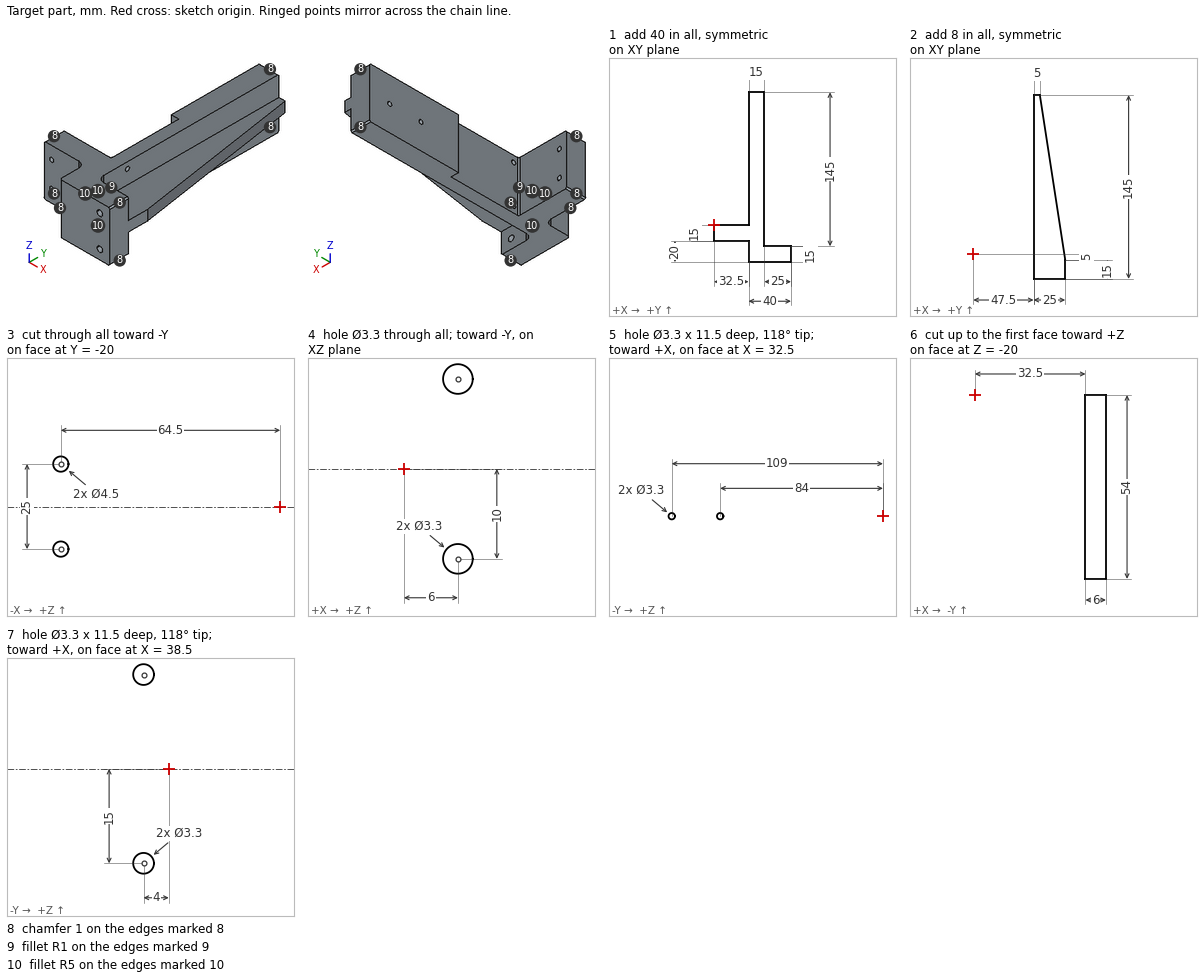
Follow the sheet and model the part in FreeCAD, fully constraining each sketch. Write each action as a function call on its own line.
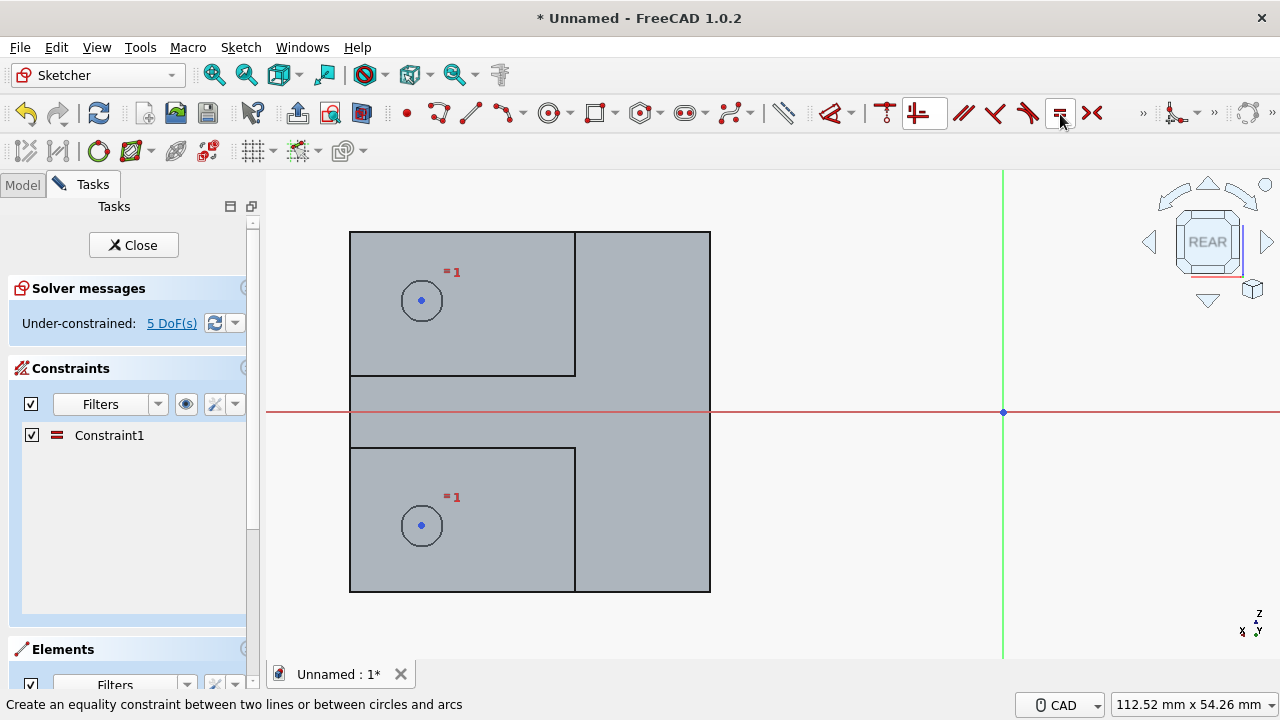
click(422, 301)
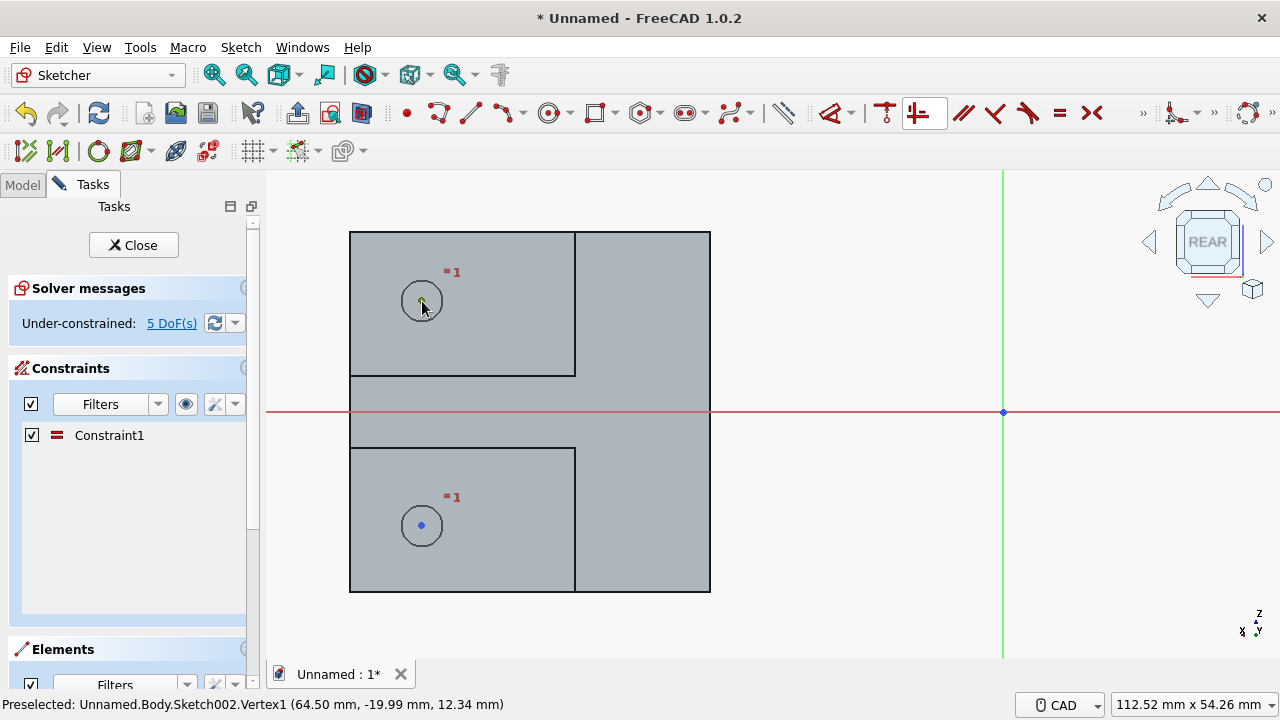
click(422, 526)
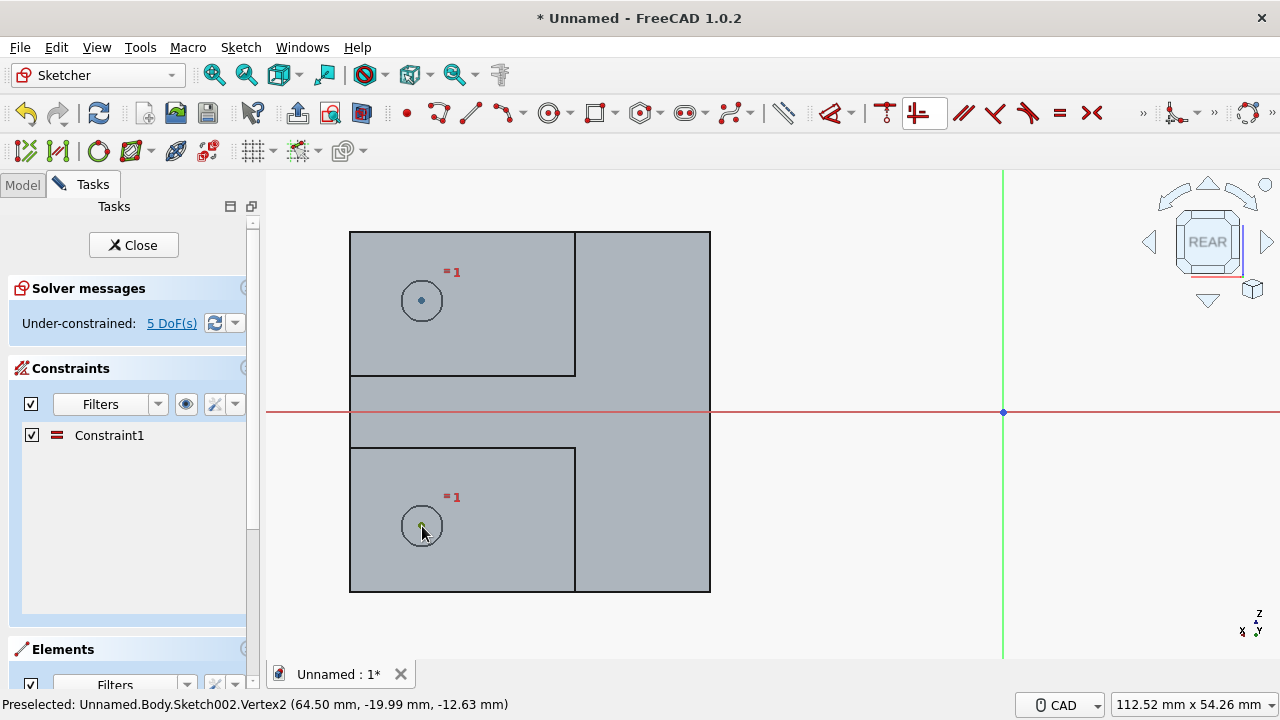
click(353, 412)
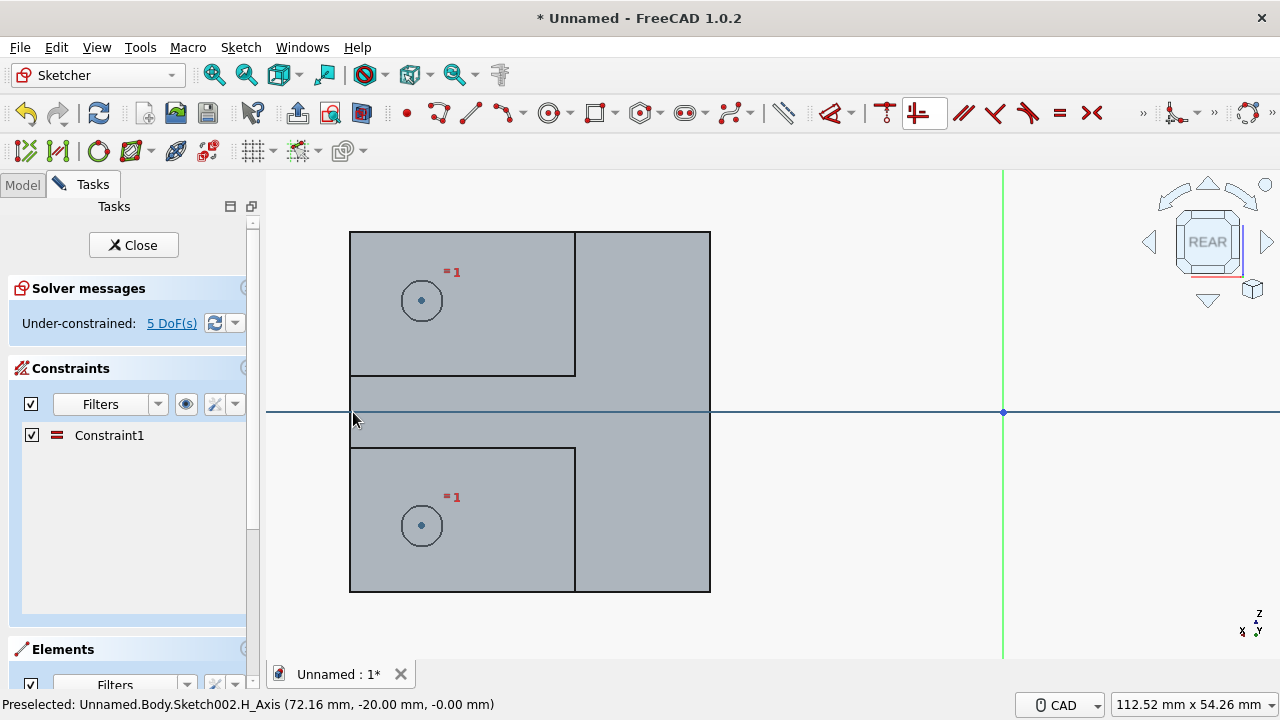
key(s)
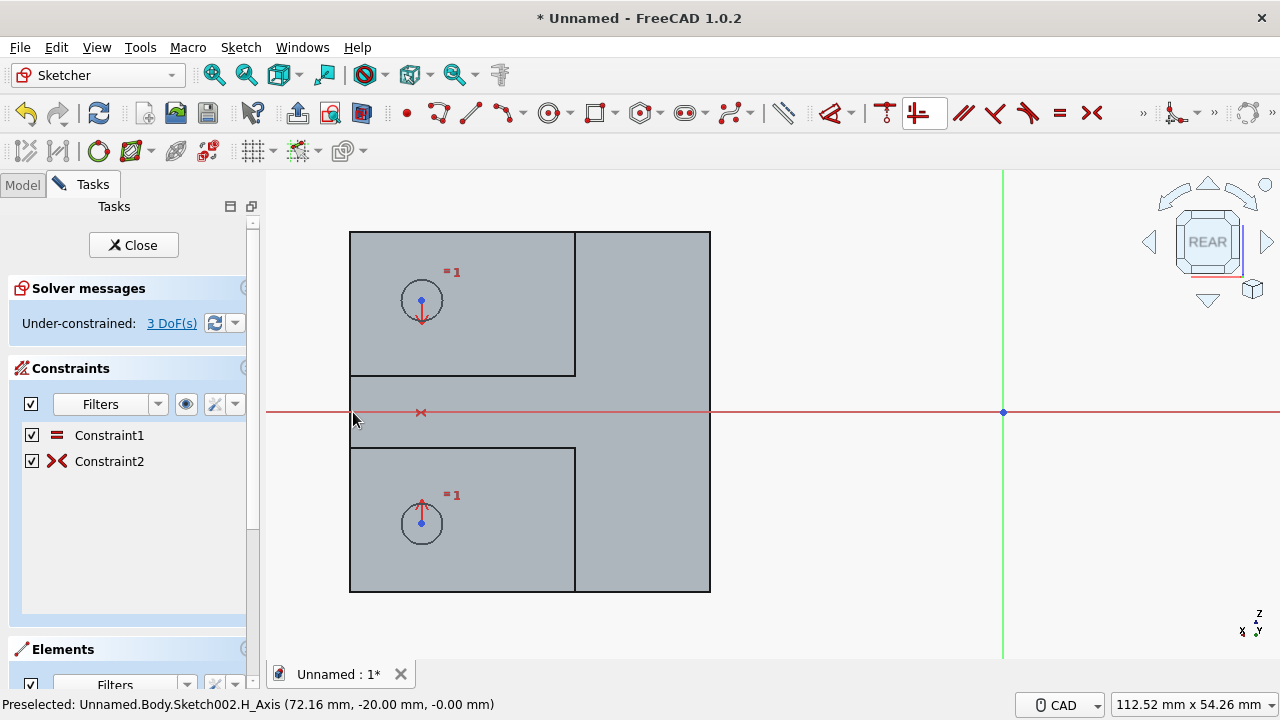
click(830, 114)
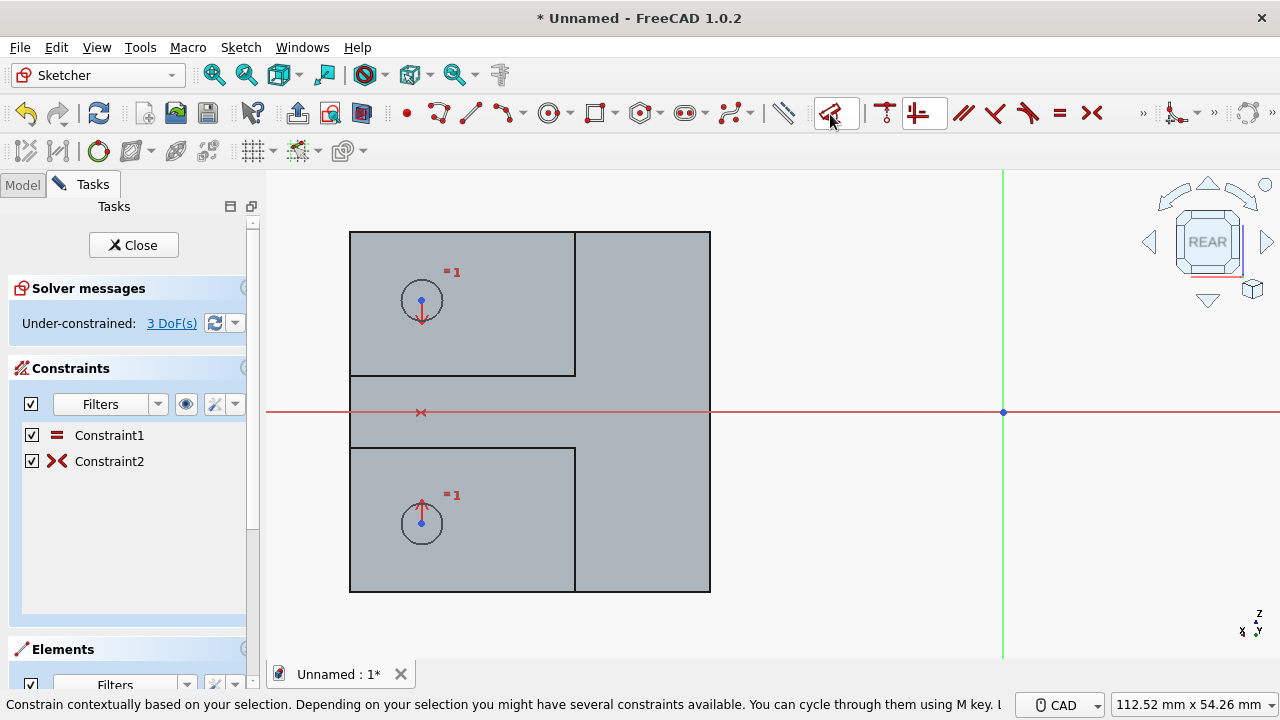
click(436, 286)
click(458, 263)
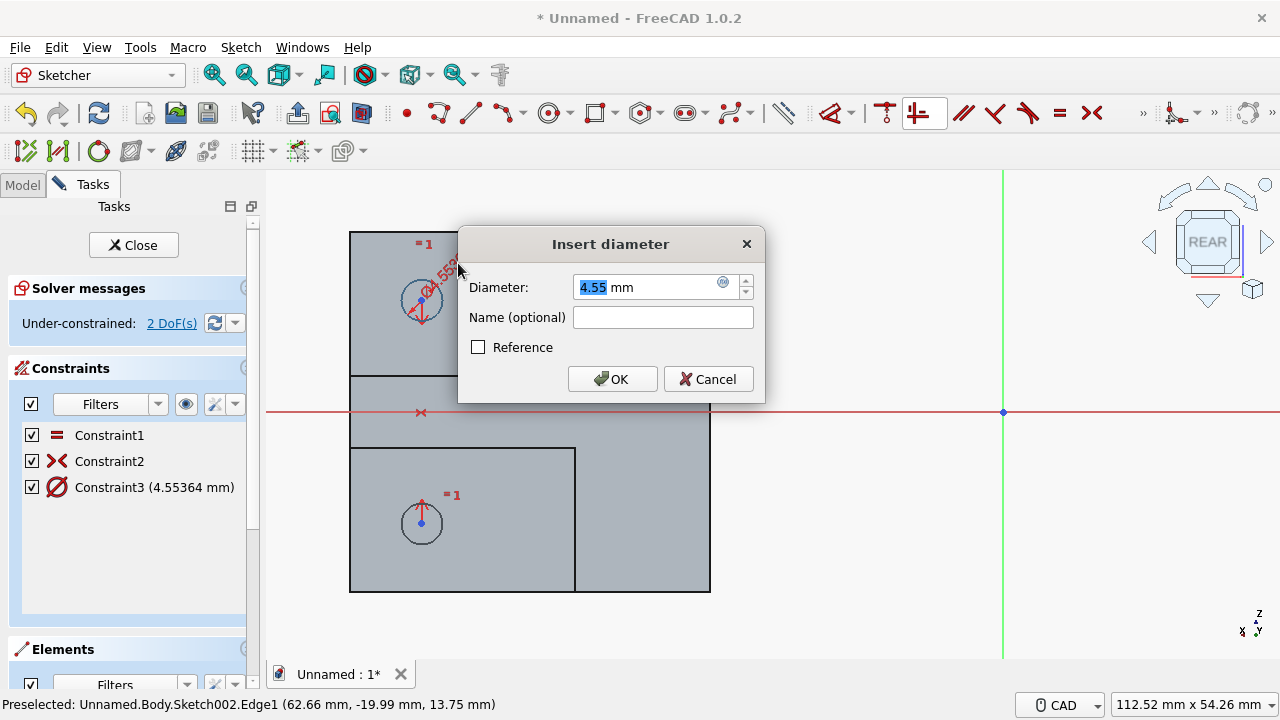
text(4.5)
key(Return)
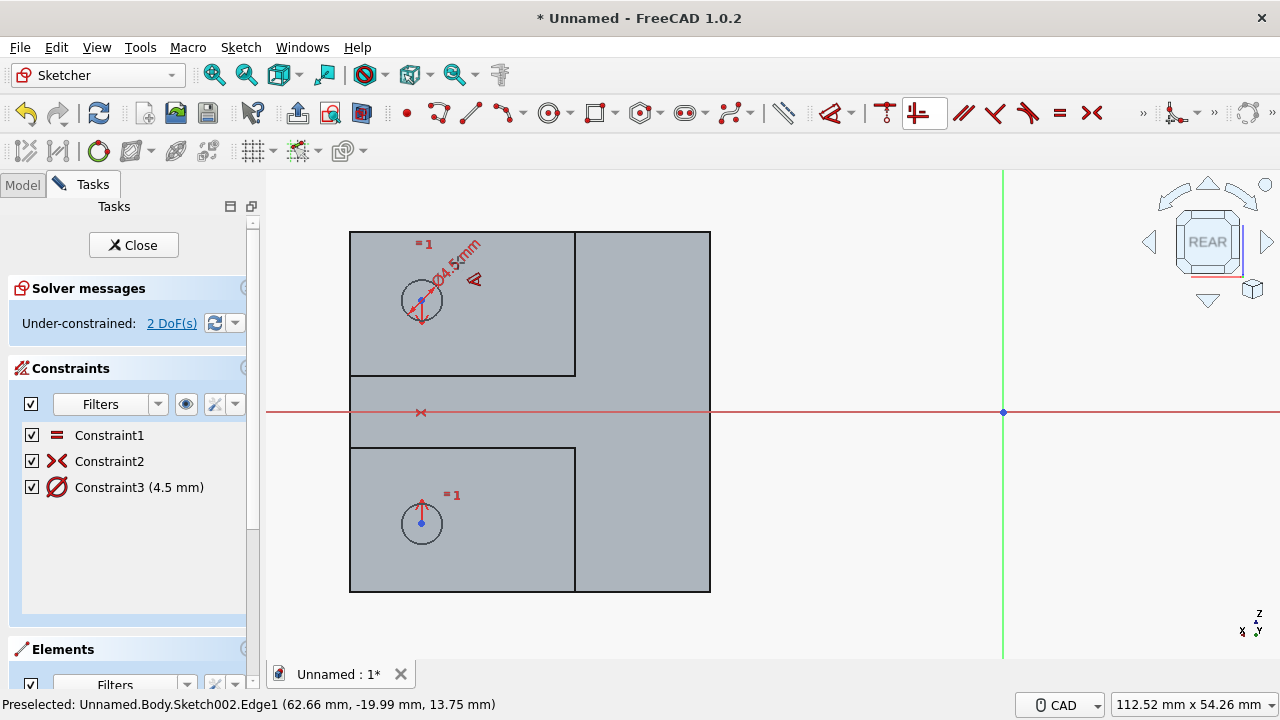
click(422, 300)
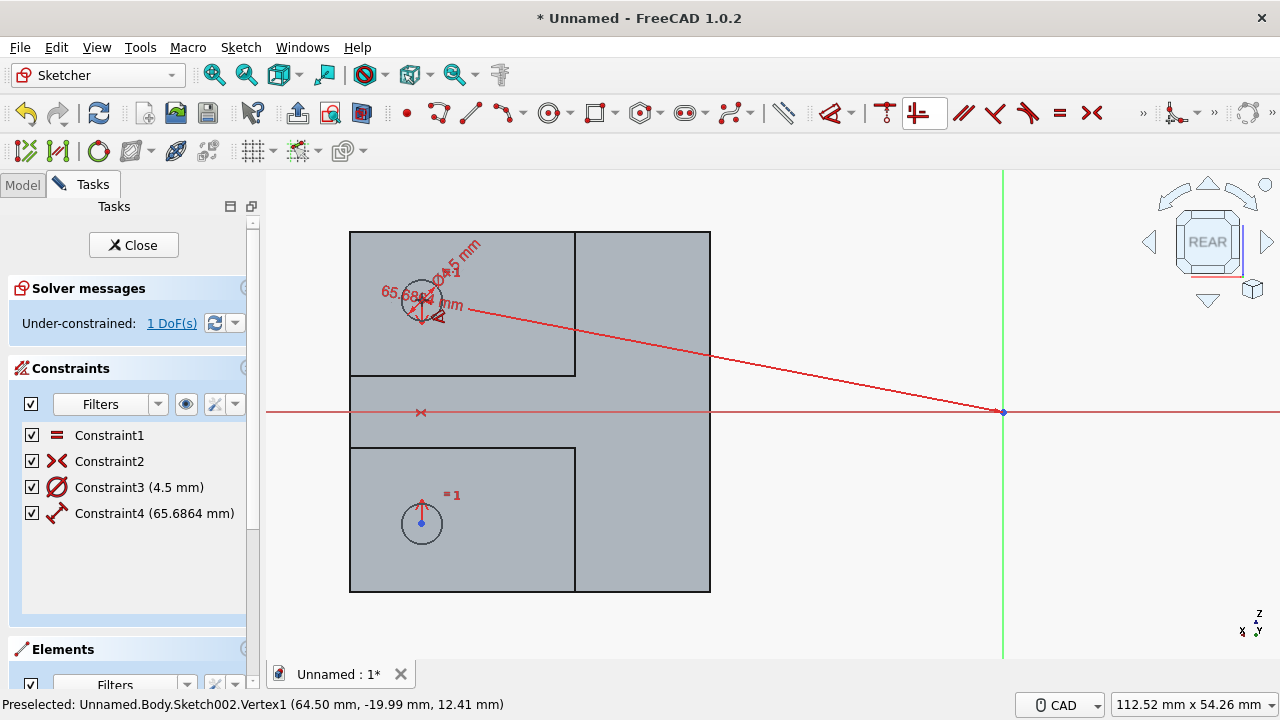
click(422, 524)
click(388, 361)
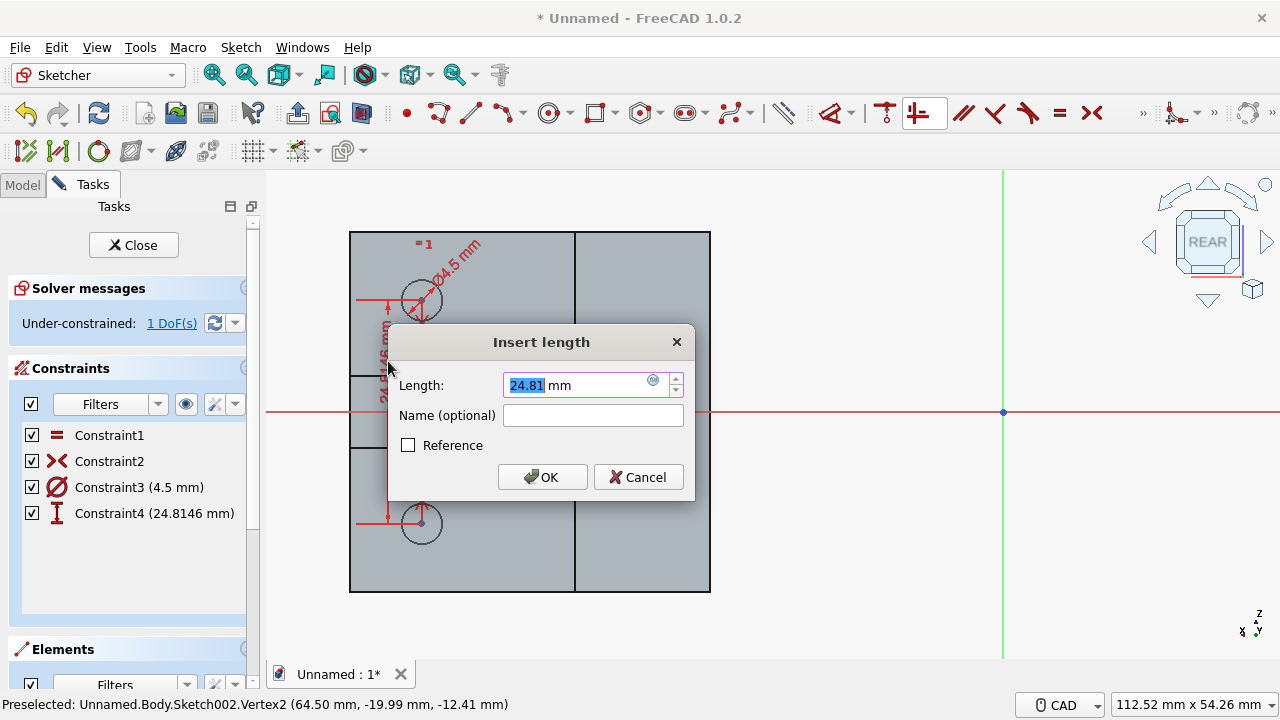
text(25)
key(Return)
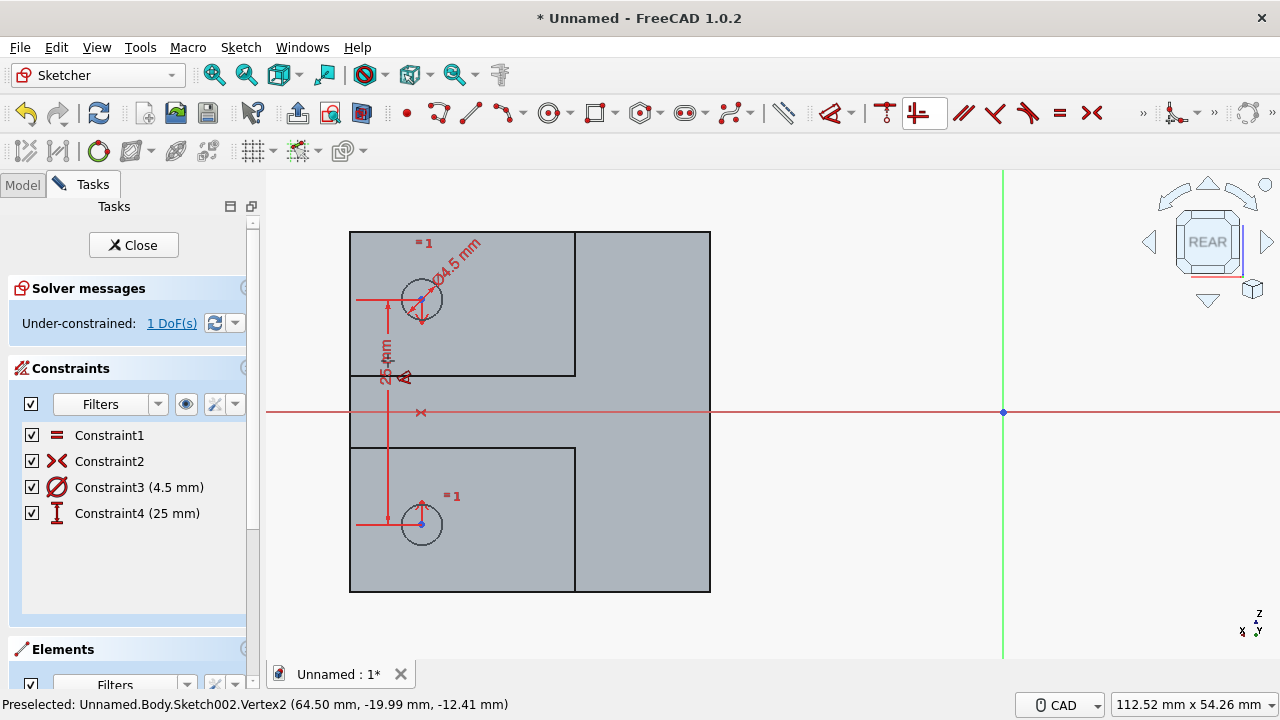
click(422, 300)
click(713, 266)